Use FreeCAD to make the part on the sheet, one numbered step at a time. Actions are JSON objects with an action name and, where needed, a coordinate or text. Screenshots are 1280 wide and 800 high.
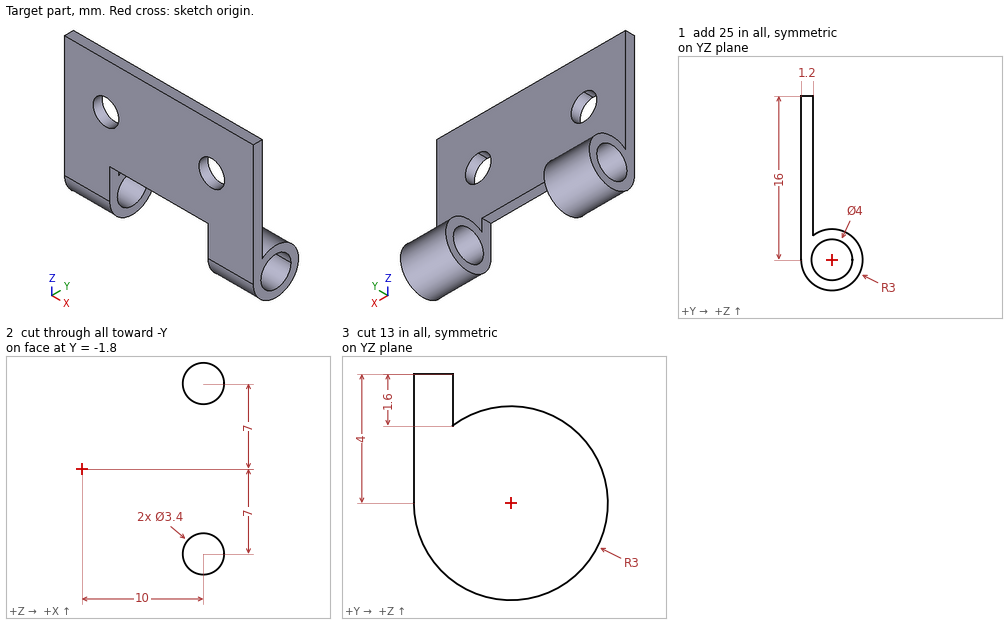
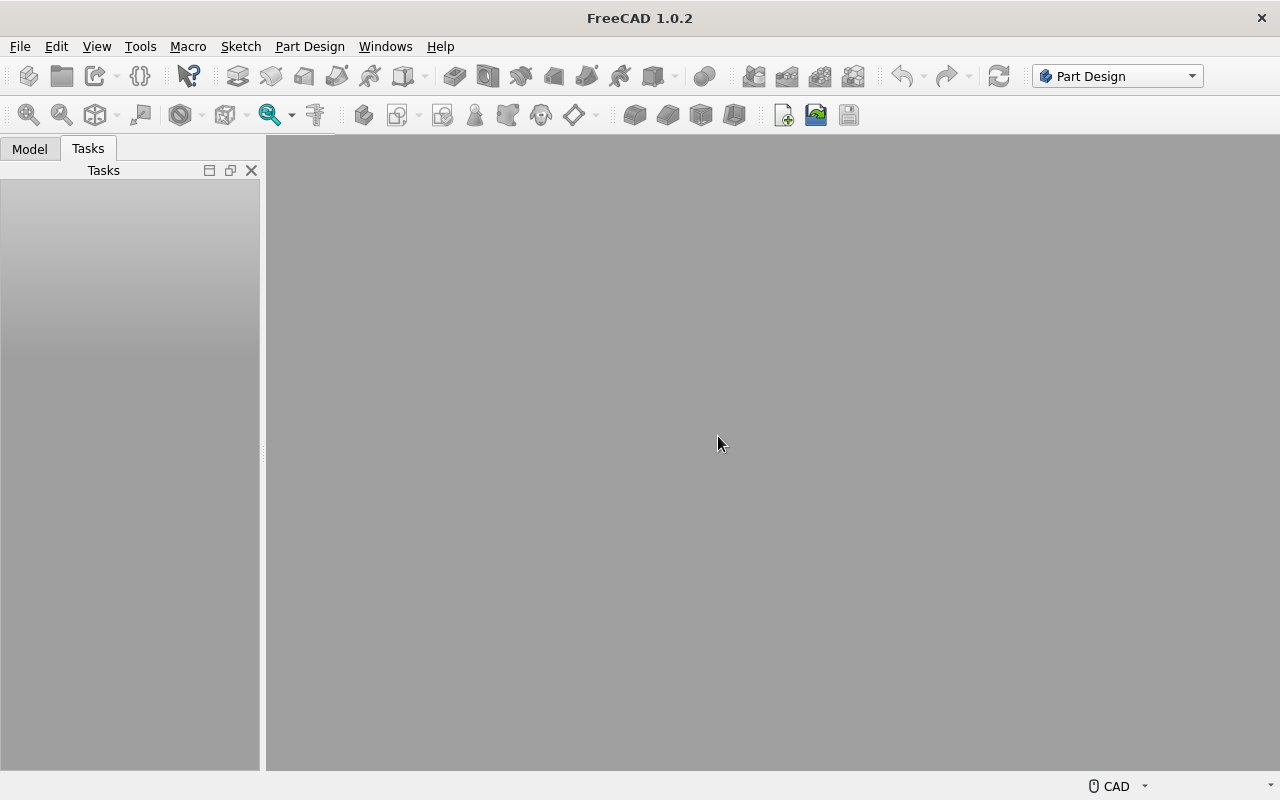
{"action": "left_click", "coordinate": [783, 116]}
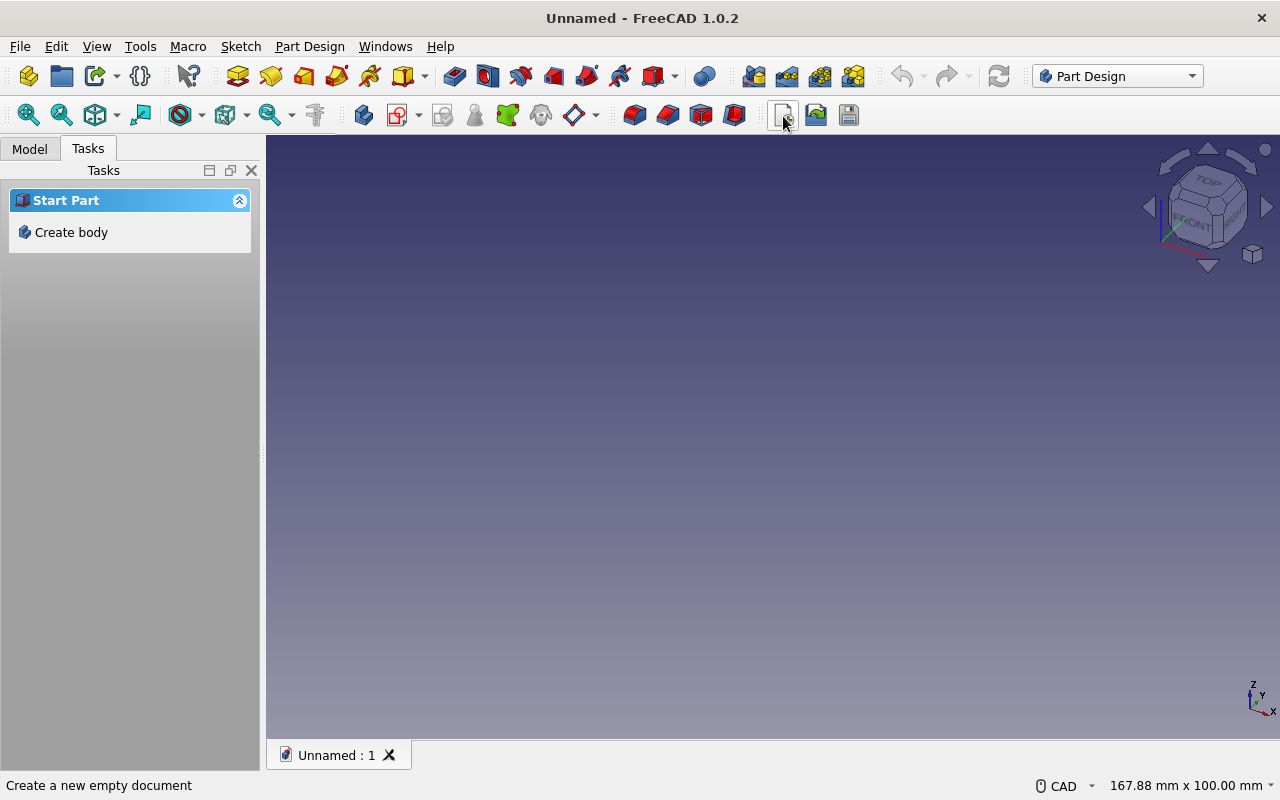
{"action": "left_click", "coordinate": [396, 116]}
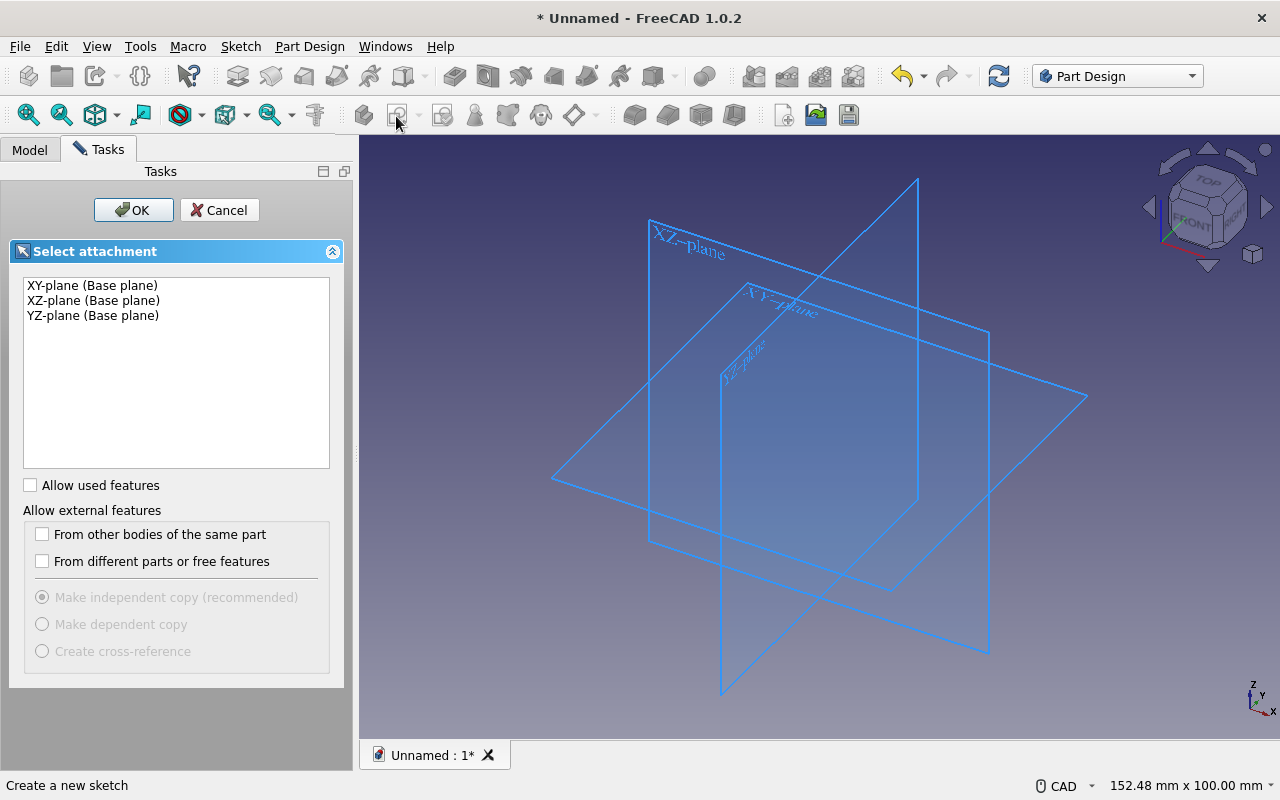
{"action": "left_click", "coordinate": [84, 316]}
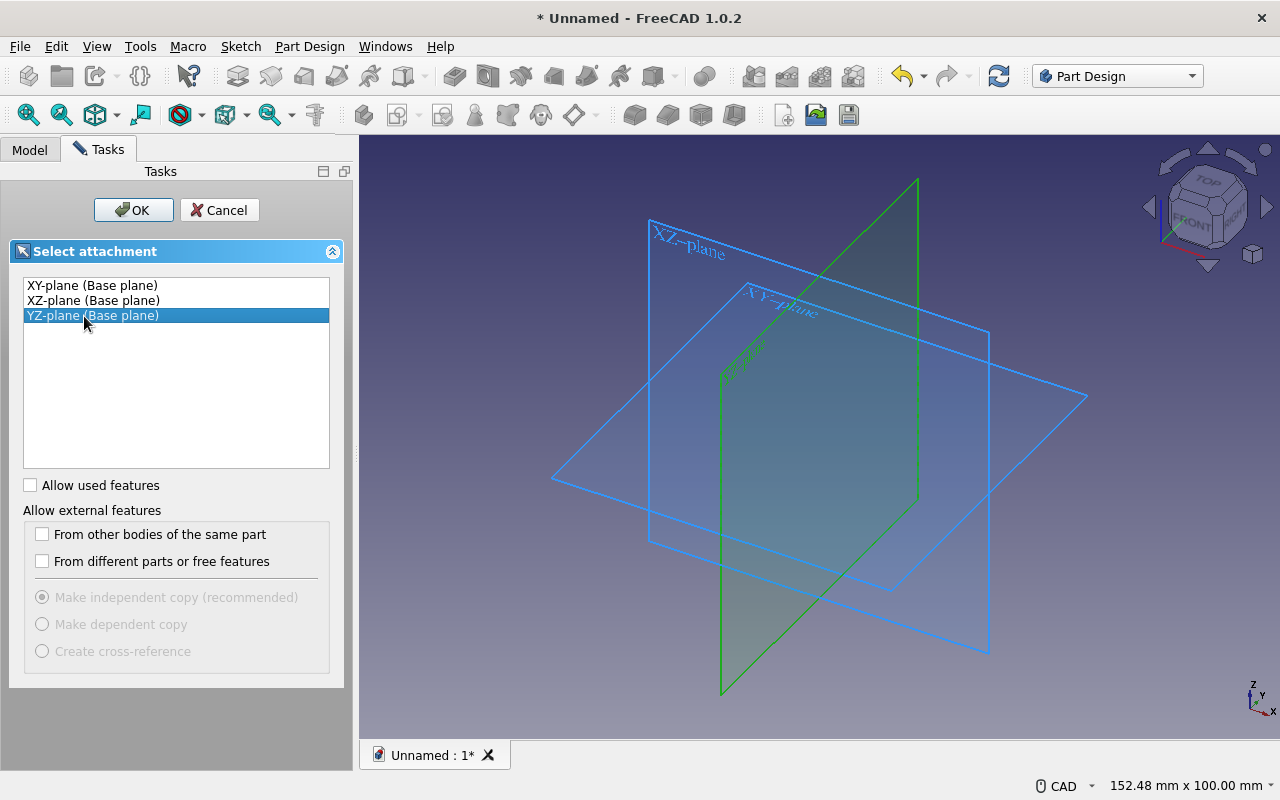
{"action": "left_click", "coordinate": [134, 210]}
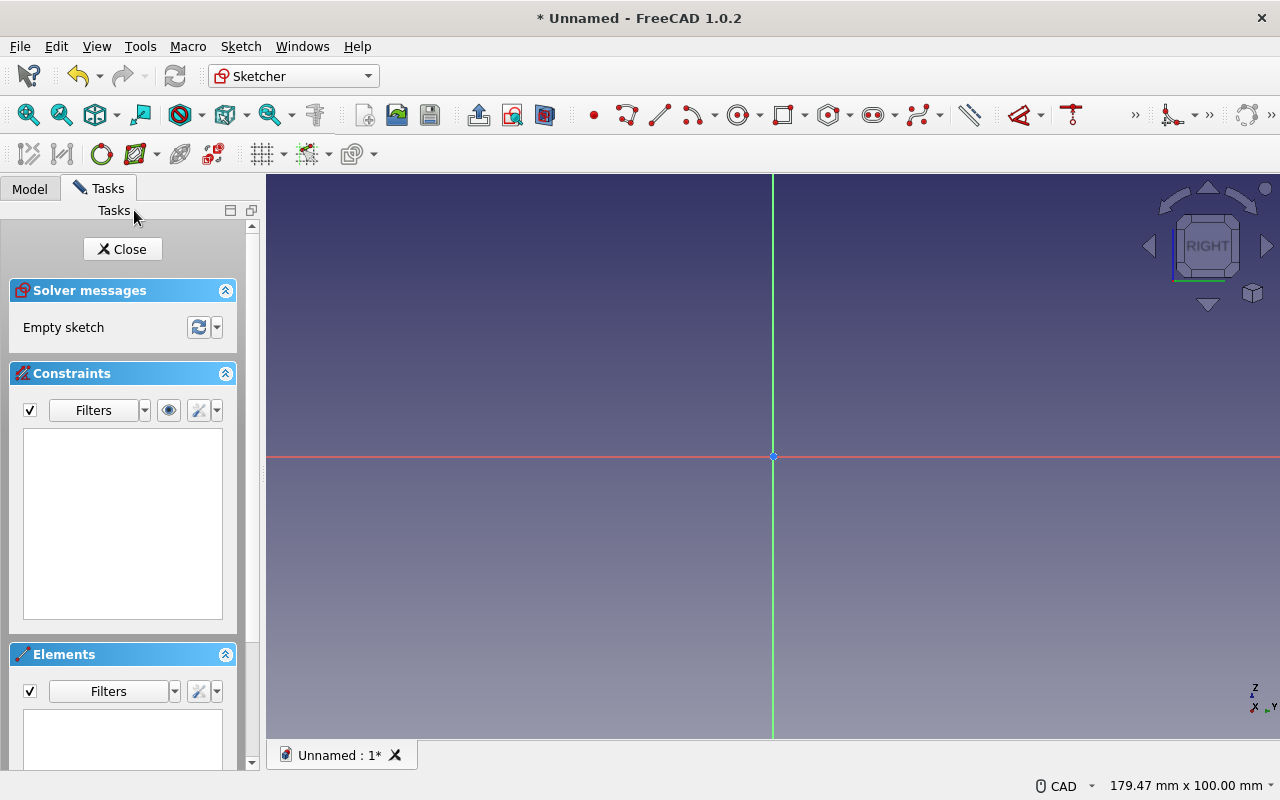
{"action": "scroll", "coordinate": [801, 400], "scroll_direction": "up", "scroll_amount": 6}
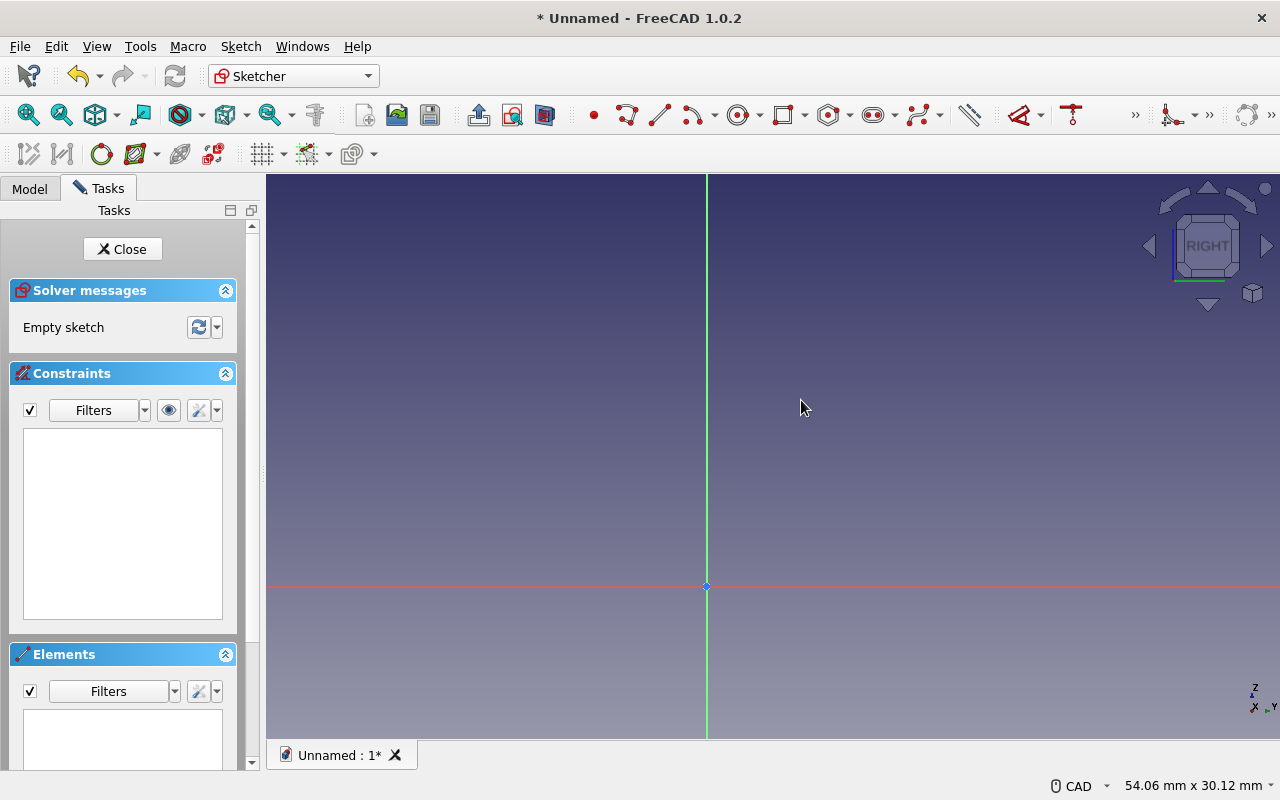
{"action": "left_click", "coordinate": [627, 116]}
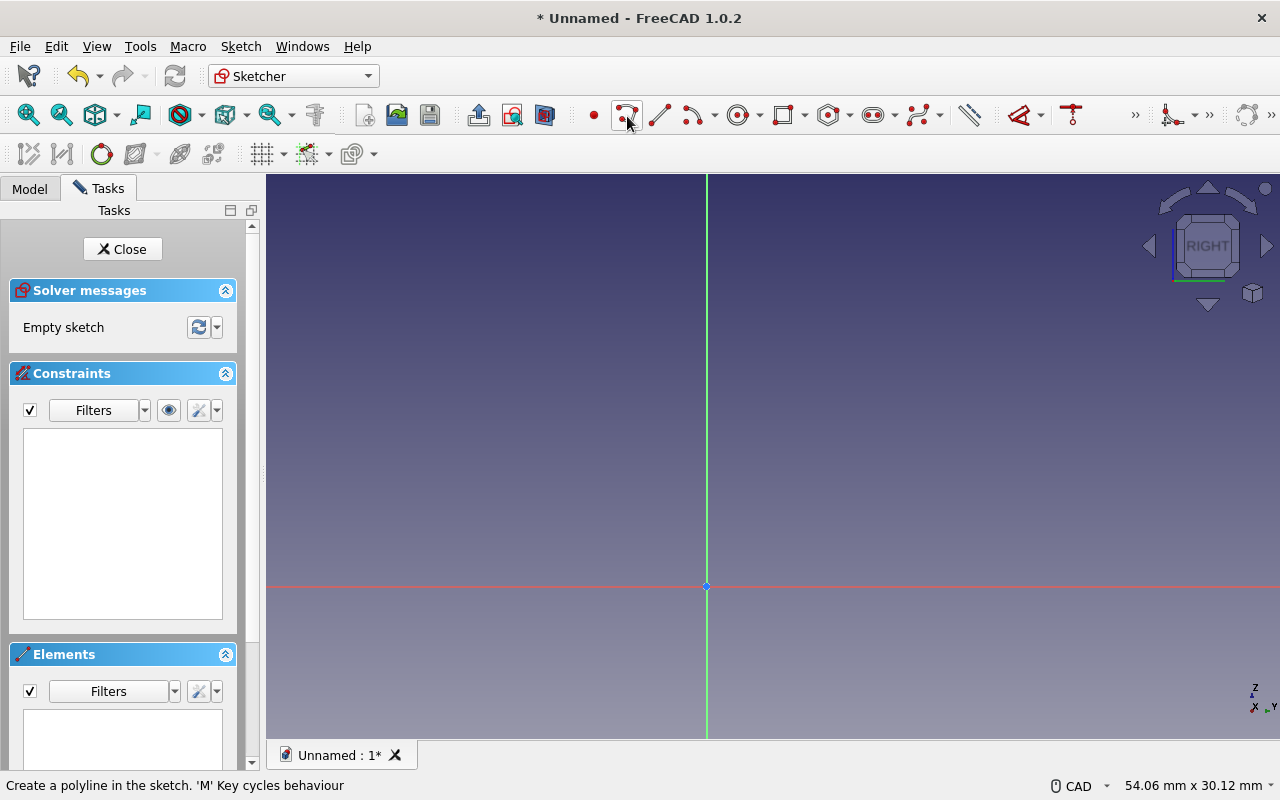
{"action": "left_click", "coordinate": [673, 542]}
{"action": "left_click", "coordinate": [673, 287]}
{"action": "left_click", "coordinate": [651, 287]}
{"action": "left_click", "coordinate": [651, 587]}
{"action": "right_click", "coordinate": [651, 587]}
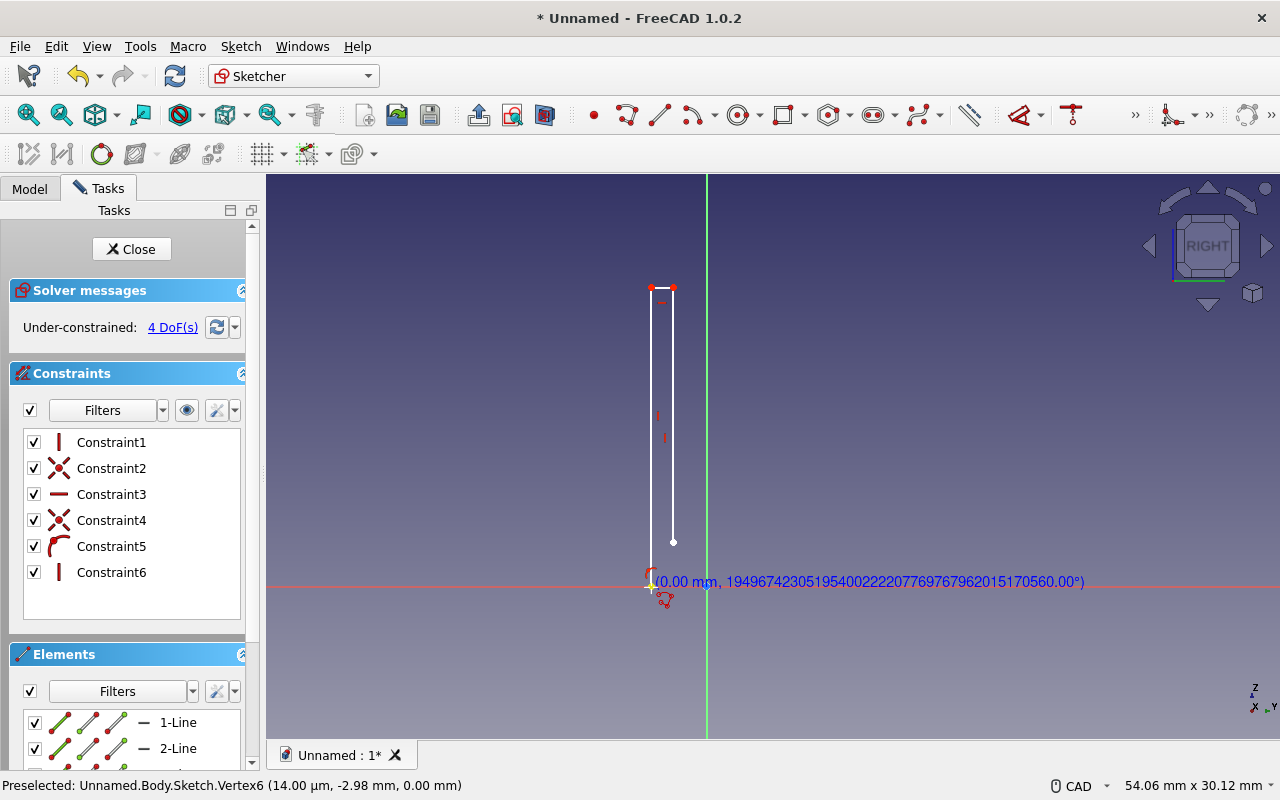
{"action": "left_click", "coordinate": [714, 116]}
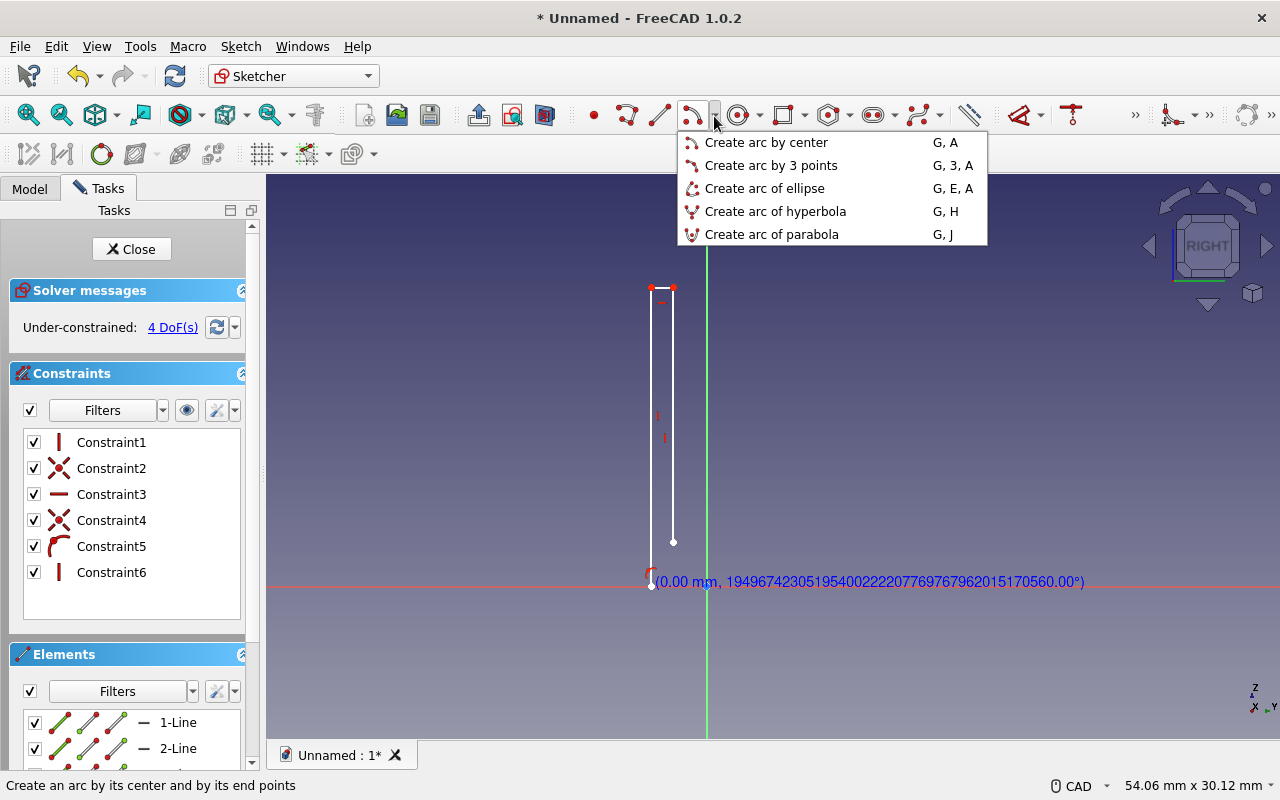
{"action": "left_click", "coordinate": [832, 166]}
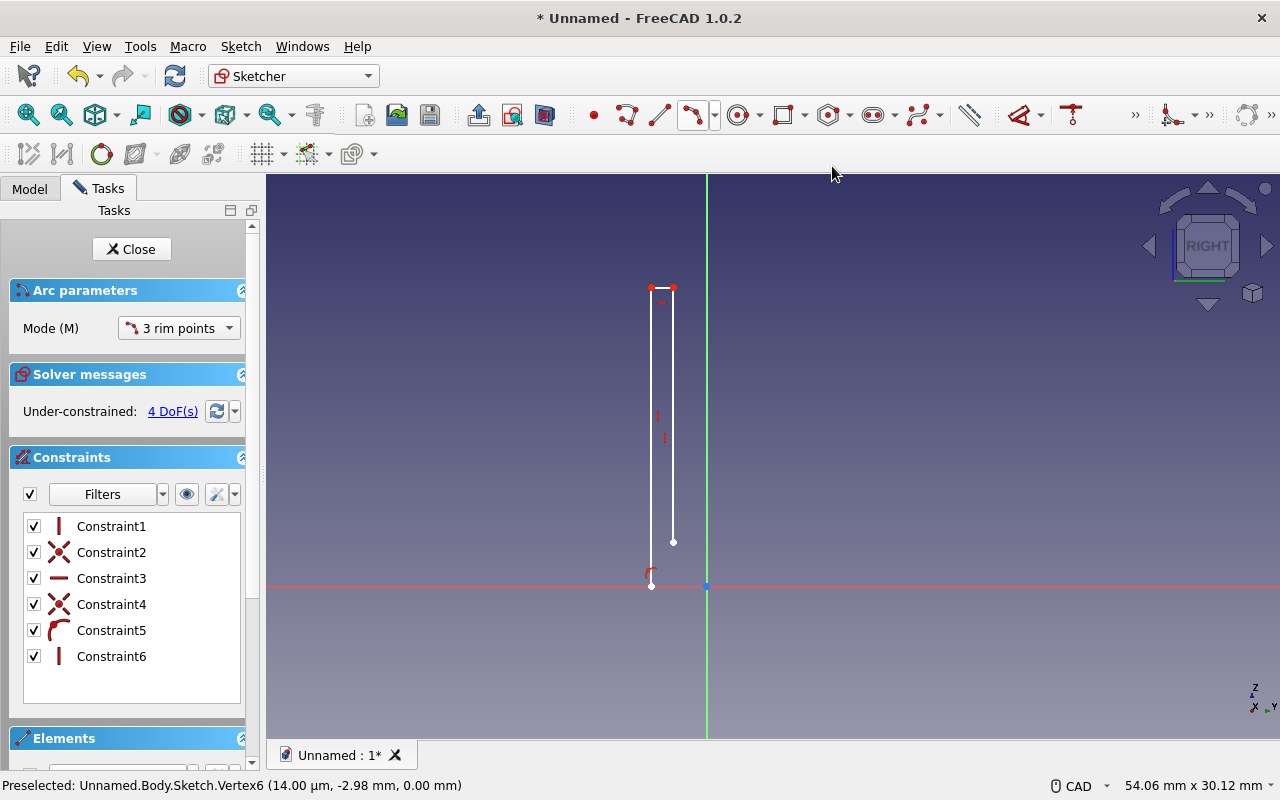
{"action": "left_click", "coordinate": [651, 587]}
{"action": "left_click", "coordinate": [673, 543]}
{"action": "left_click", "coordinate": [757, 612]}